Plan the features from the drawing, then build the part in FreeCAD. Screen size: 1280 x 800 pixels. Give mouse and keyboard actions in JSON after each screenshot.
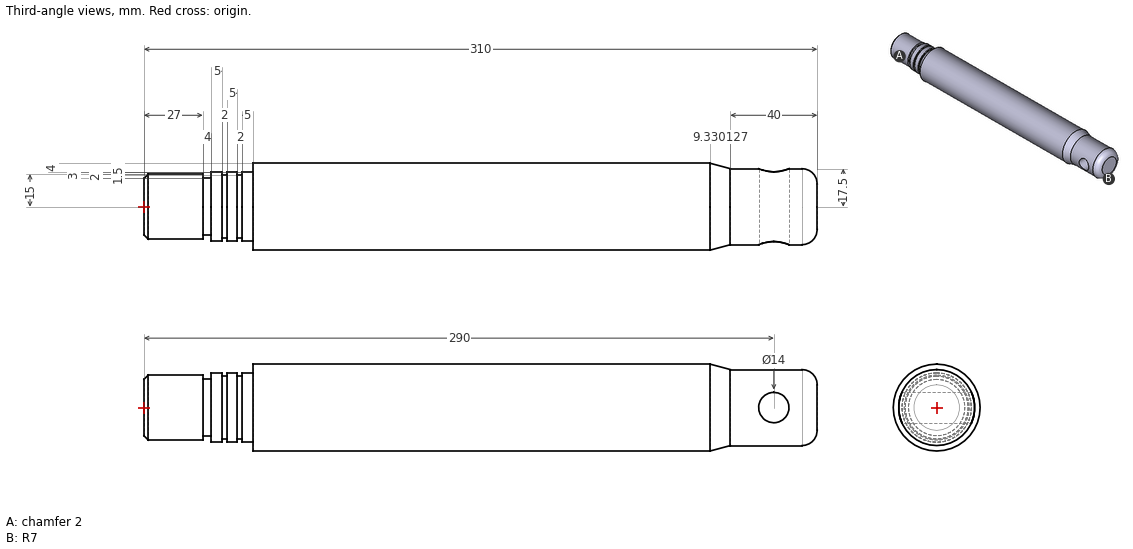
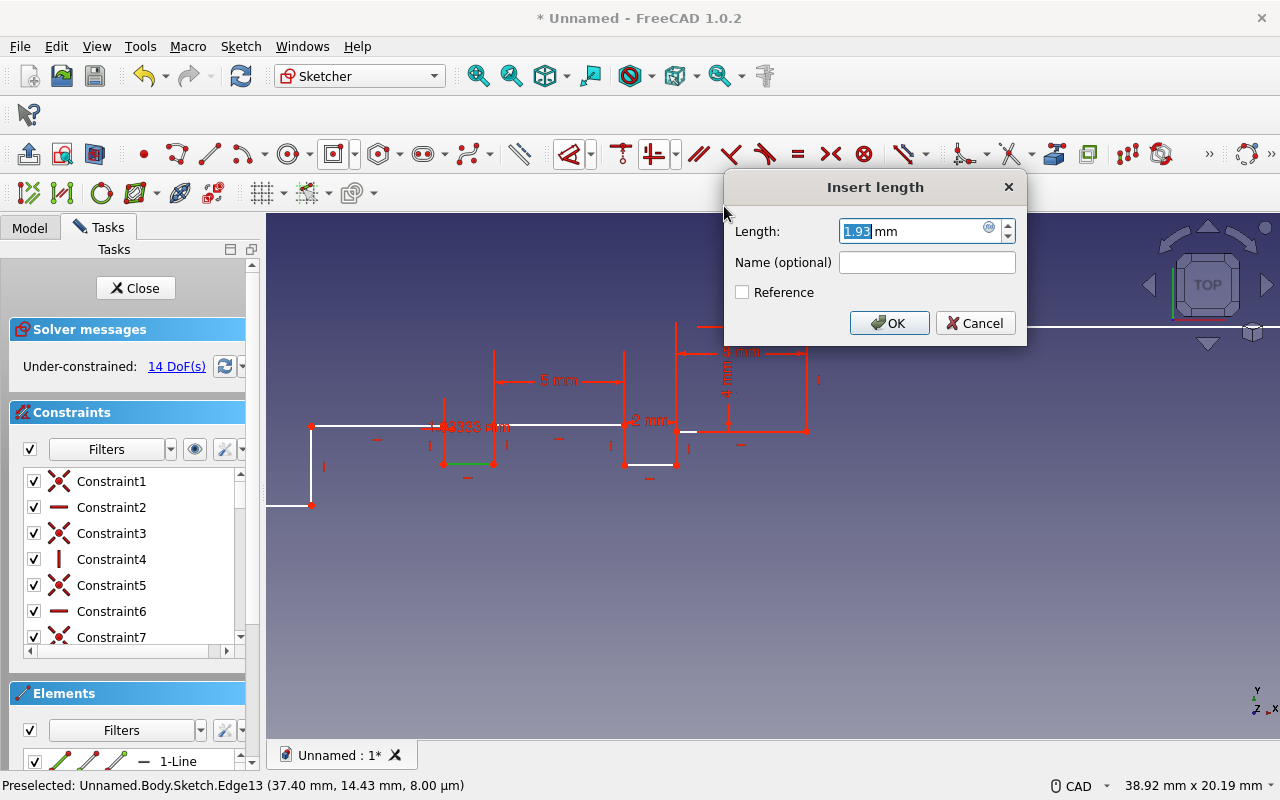
{"action": "type", "text": "2"}
{"action": "key", "text": "Return"}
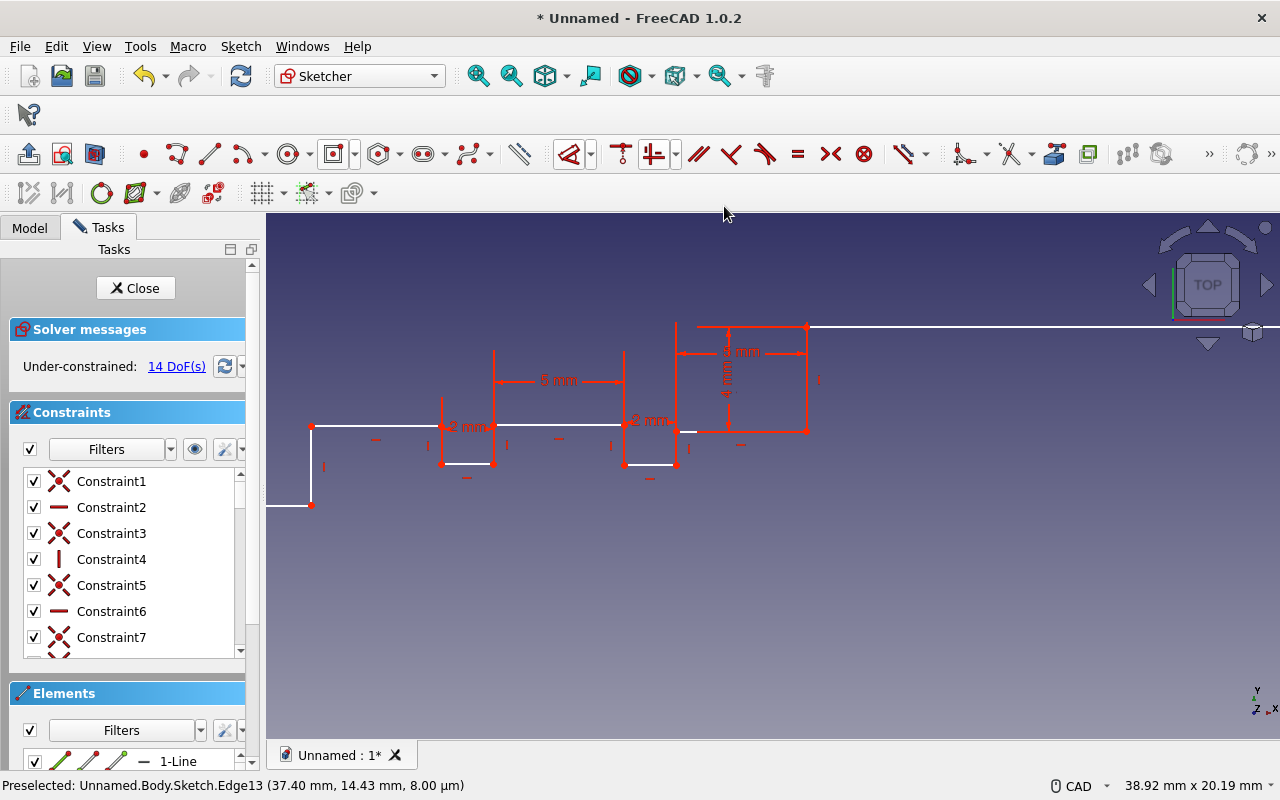
{"action": "left_click", "coordinate": [403, 426]}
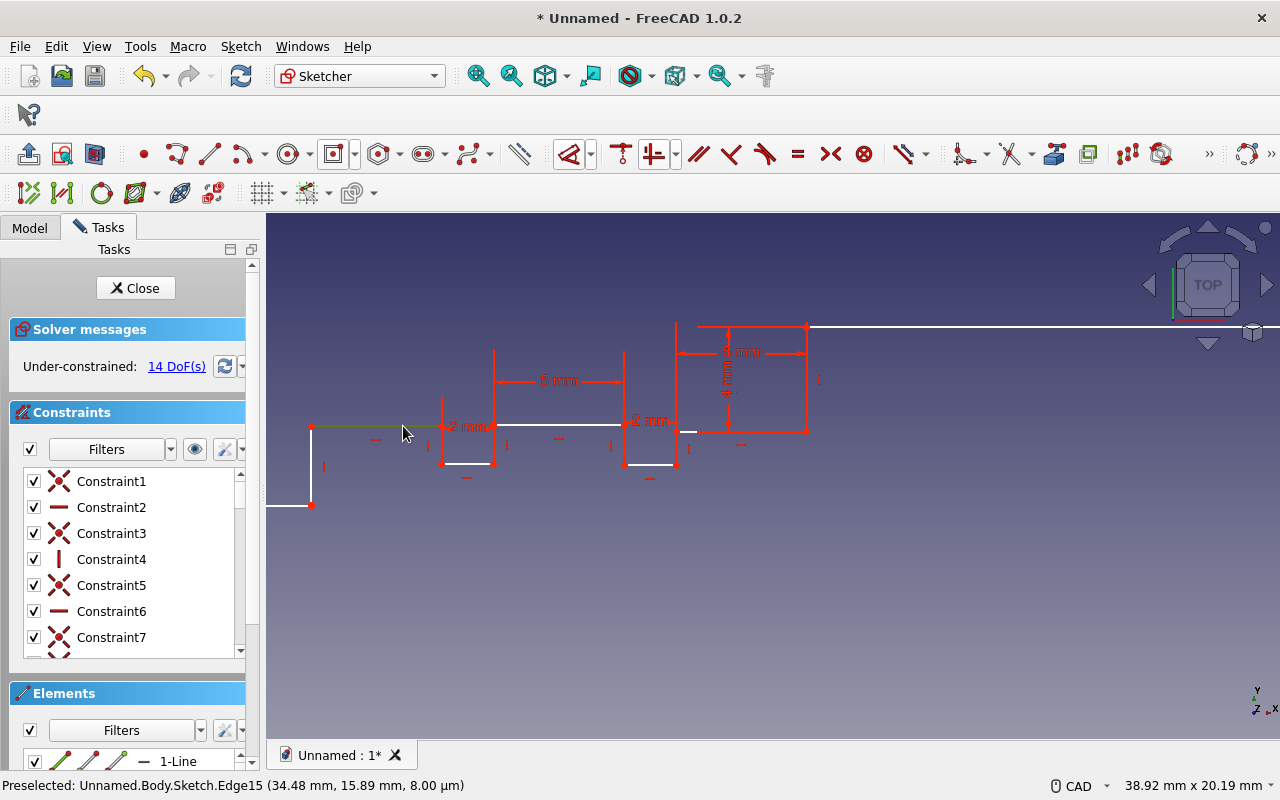
{"action": "left_click", "coordinate": [590, 154]}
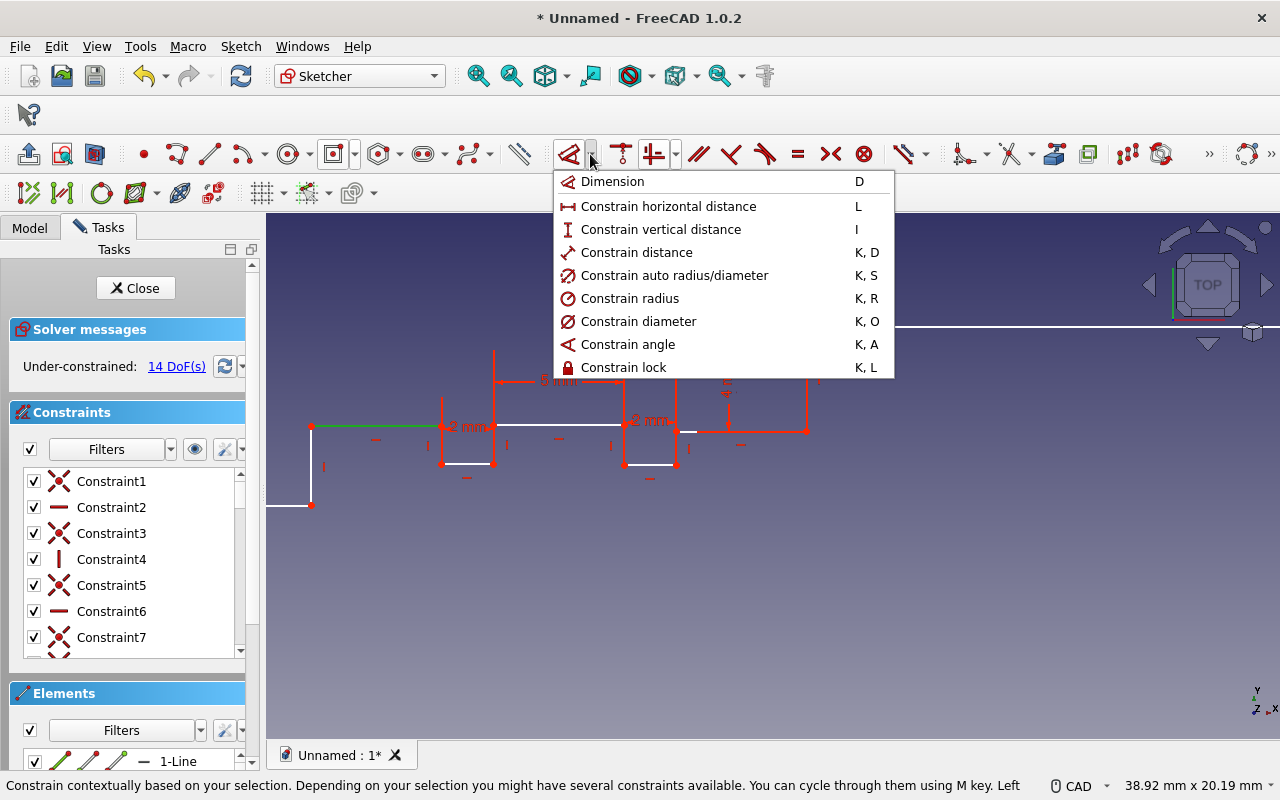
{"action": "left_click", "coordinate": [724, 206]}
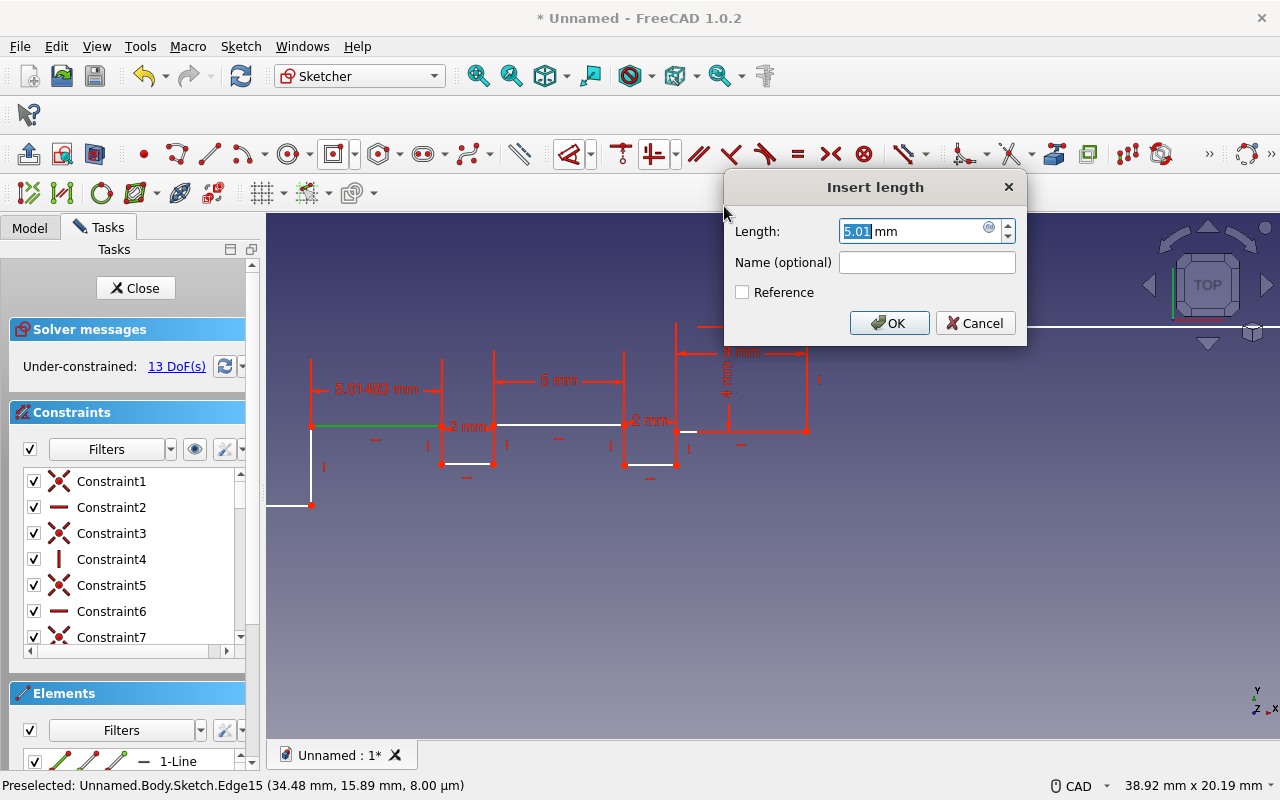
{"action": "type", "text": "5"}
{"action": "key", "text": "Return"}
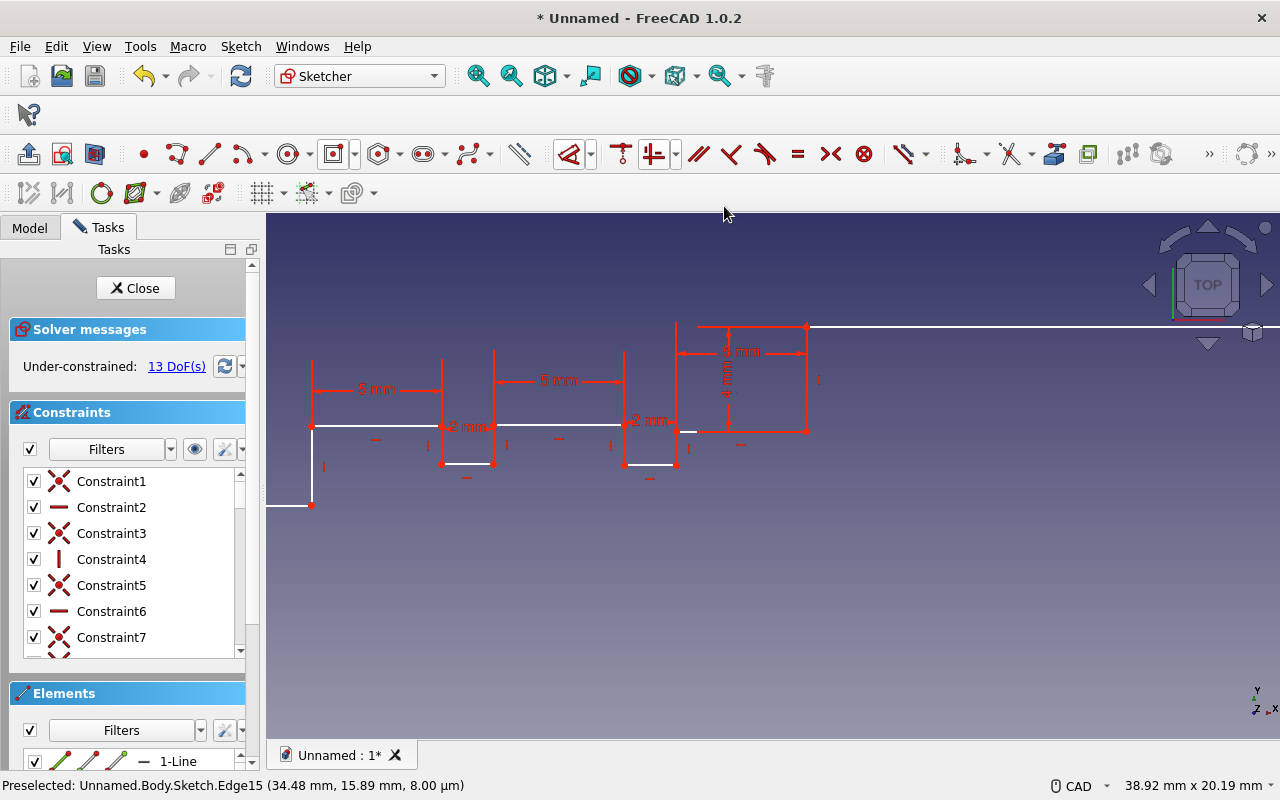
{"action": "left_click", "coordinate": [312, 450]}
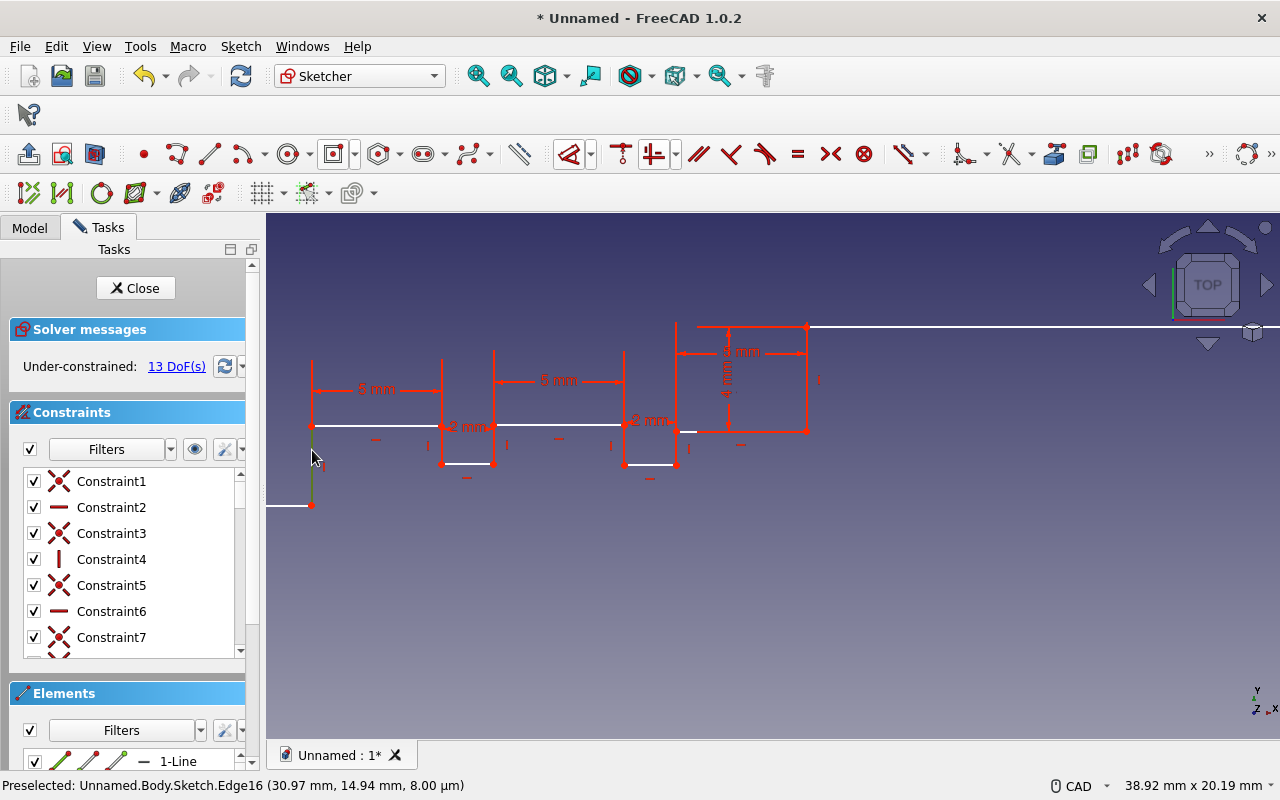
{"action": "key", "text": "i"}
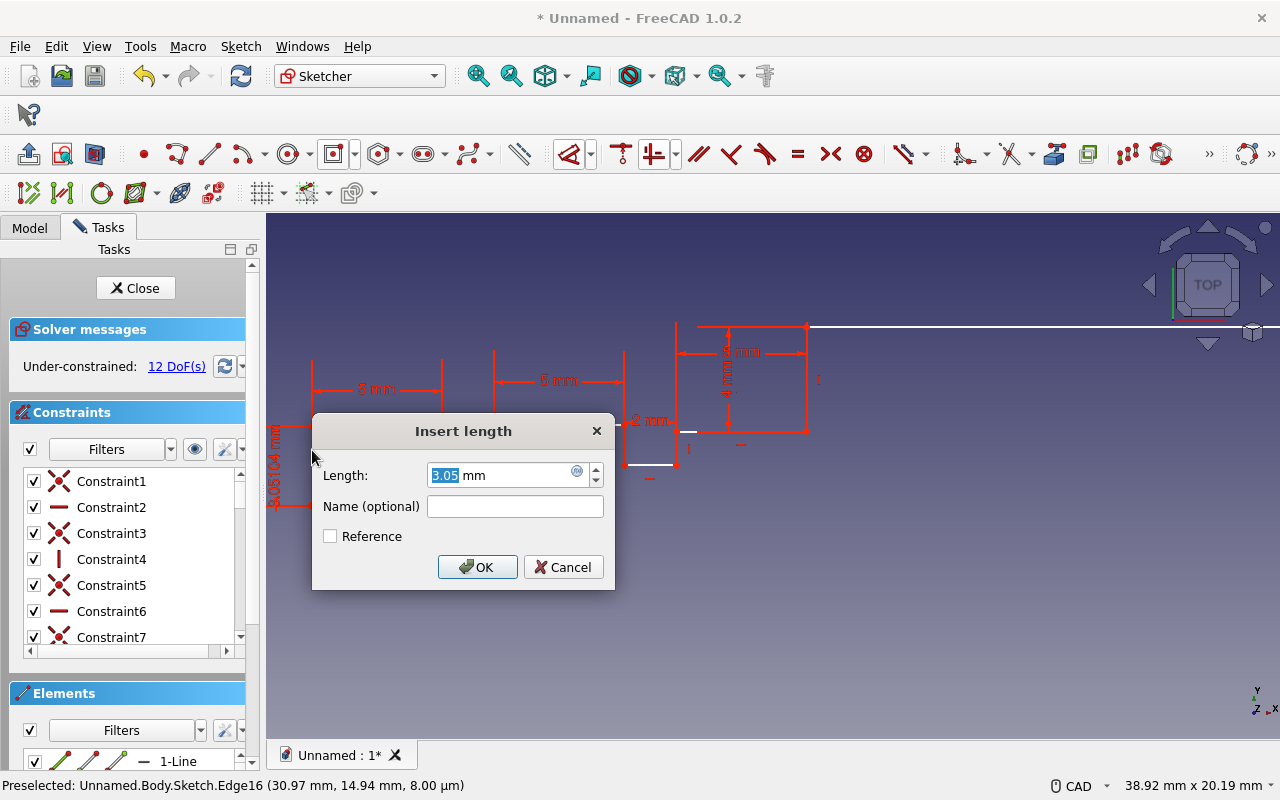
{"action": "type", "text": "3"}
{"action": "key", "text": "Return"}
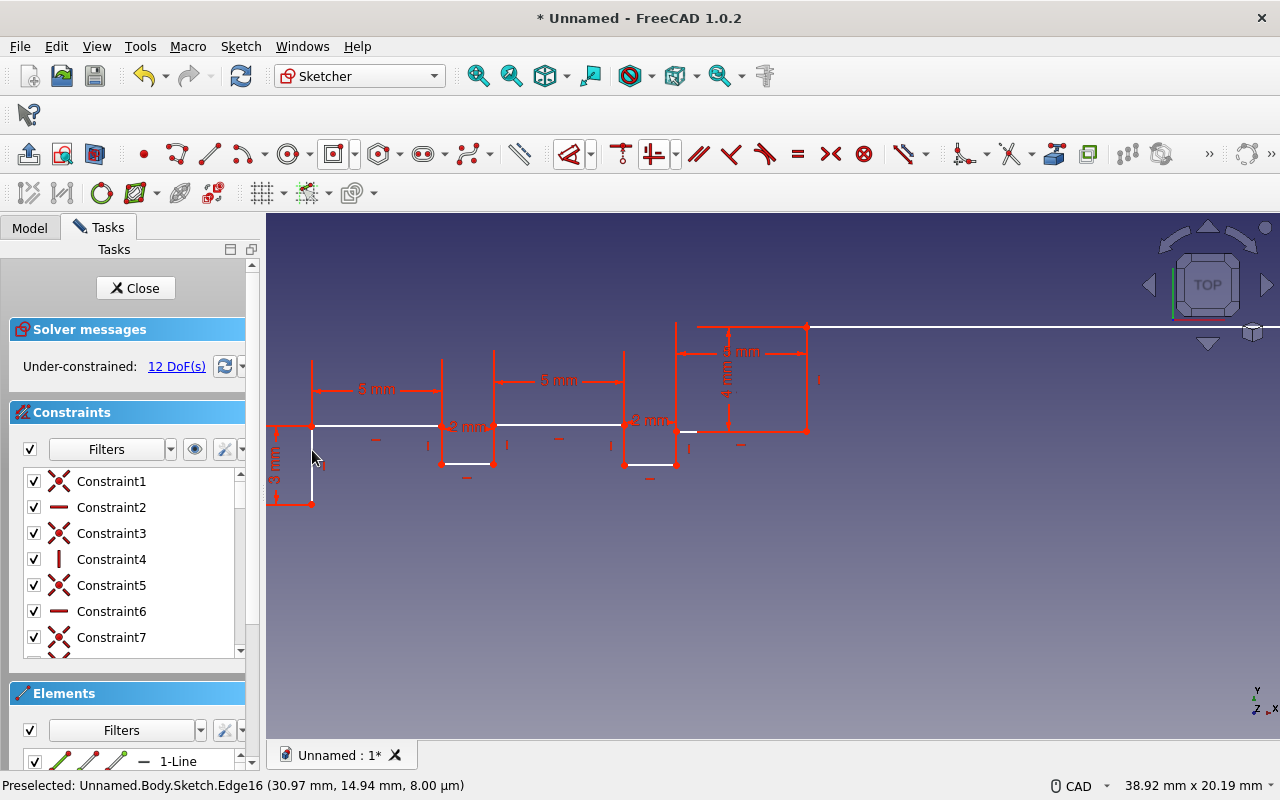
{"action": "scroll", "coordinate": [477, 468], "scroll_direction": "down", "scroll_amount": 13}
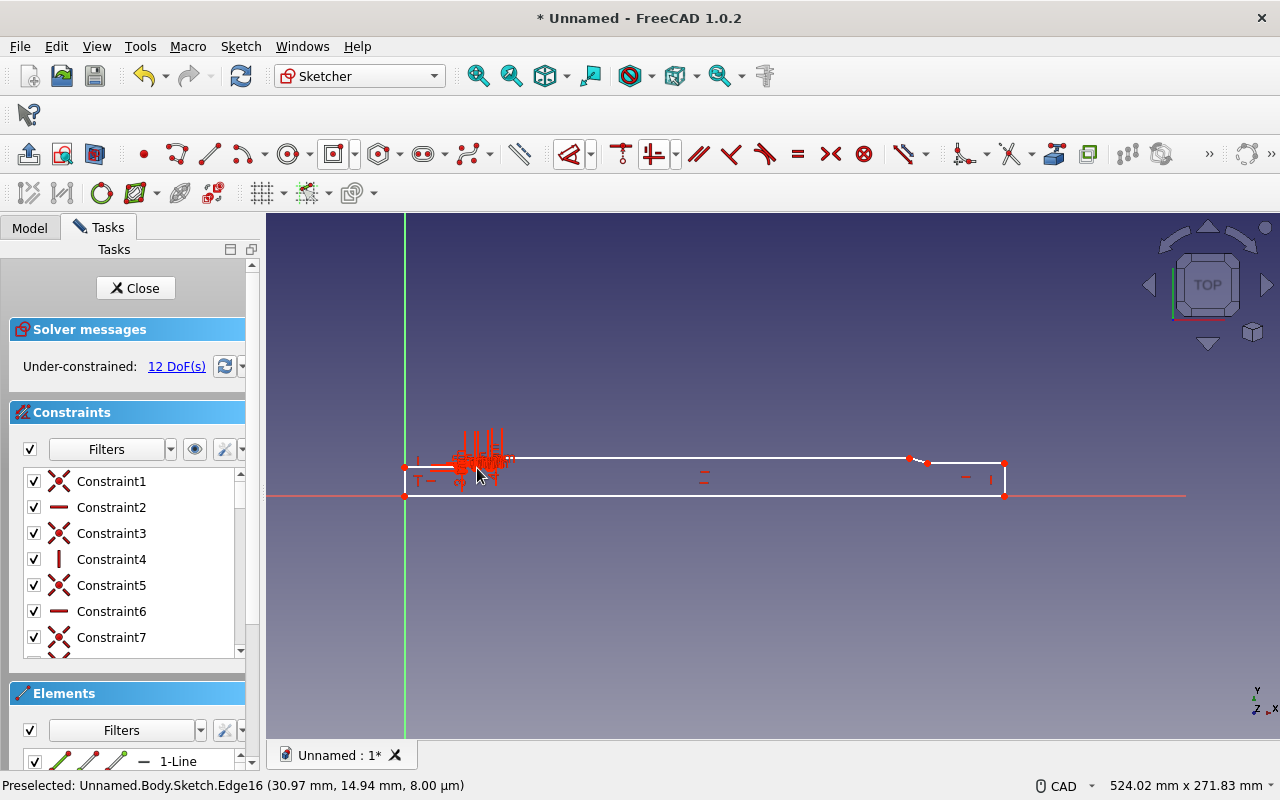
{"action": "scroll", "coordinate": [463, 471], "scroll_direction": "up", "scroll_amount": 9}